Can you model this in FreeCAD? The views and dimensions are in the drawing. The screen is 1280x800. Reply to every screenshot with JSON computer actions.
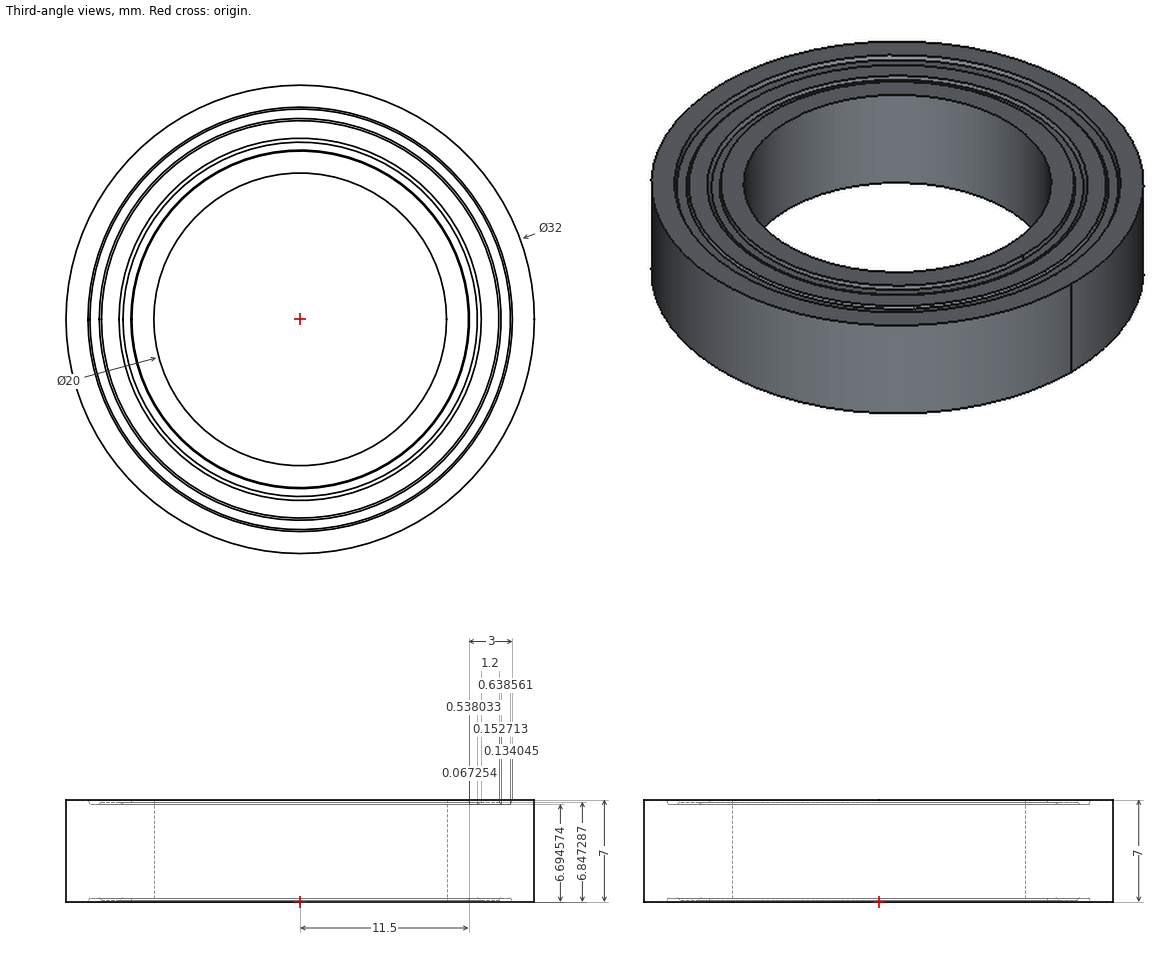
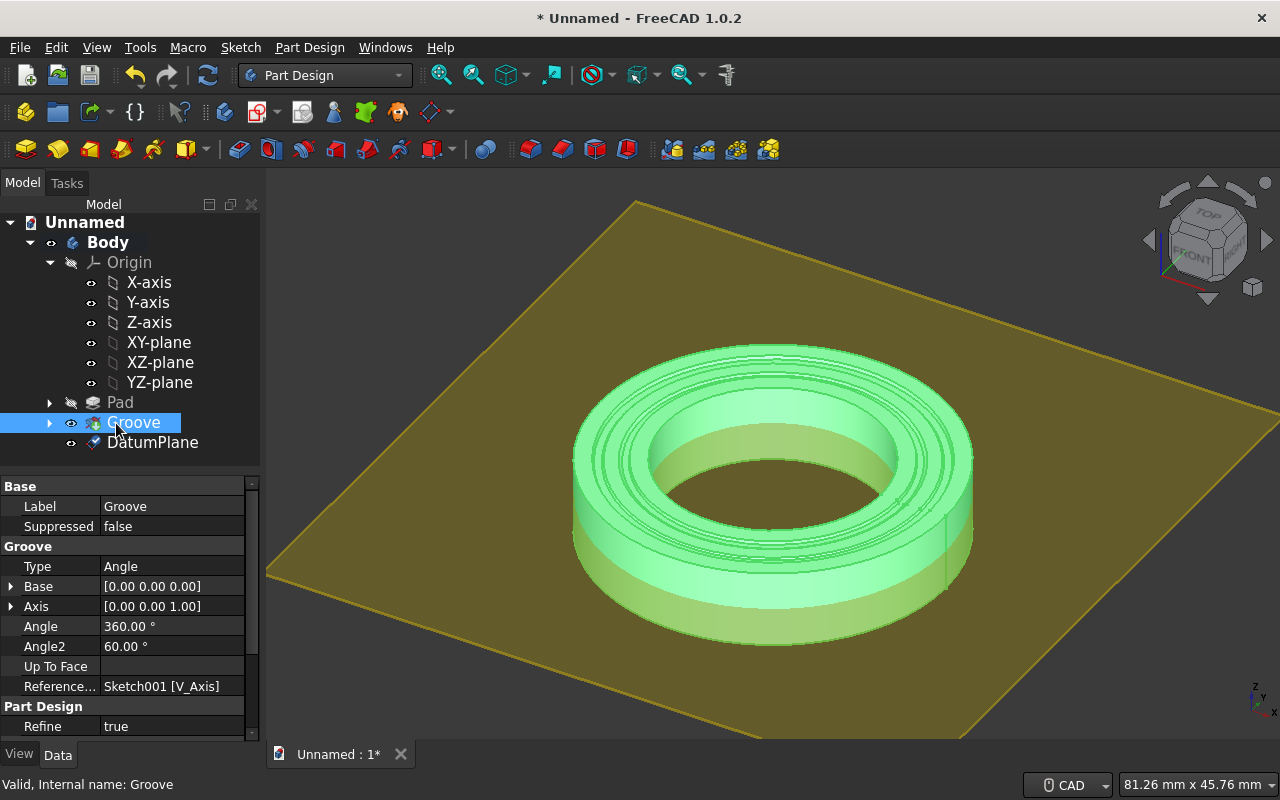
{"action": "left_click", "coordinate": [672, 150]}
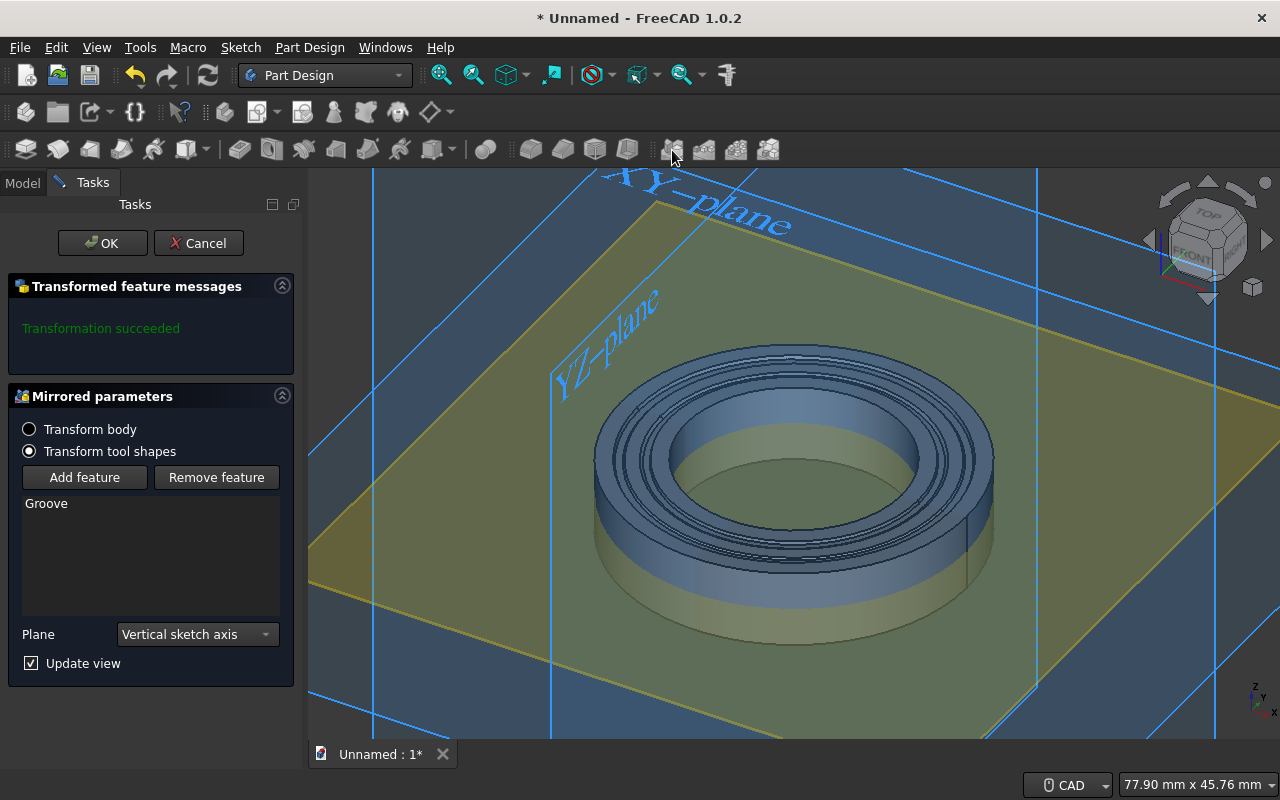
{"action": "left_click", "coordinate": [198, 634]}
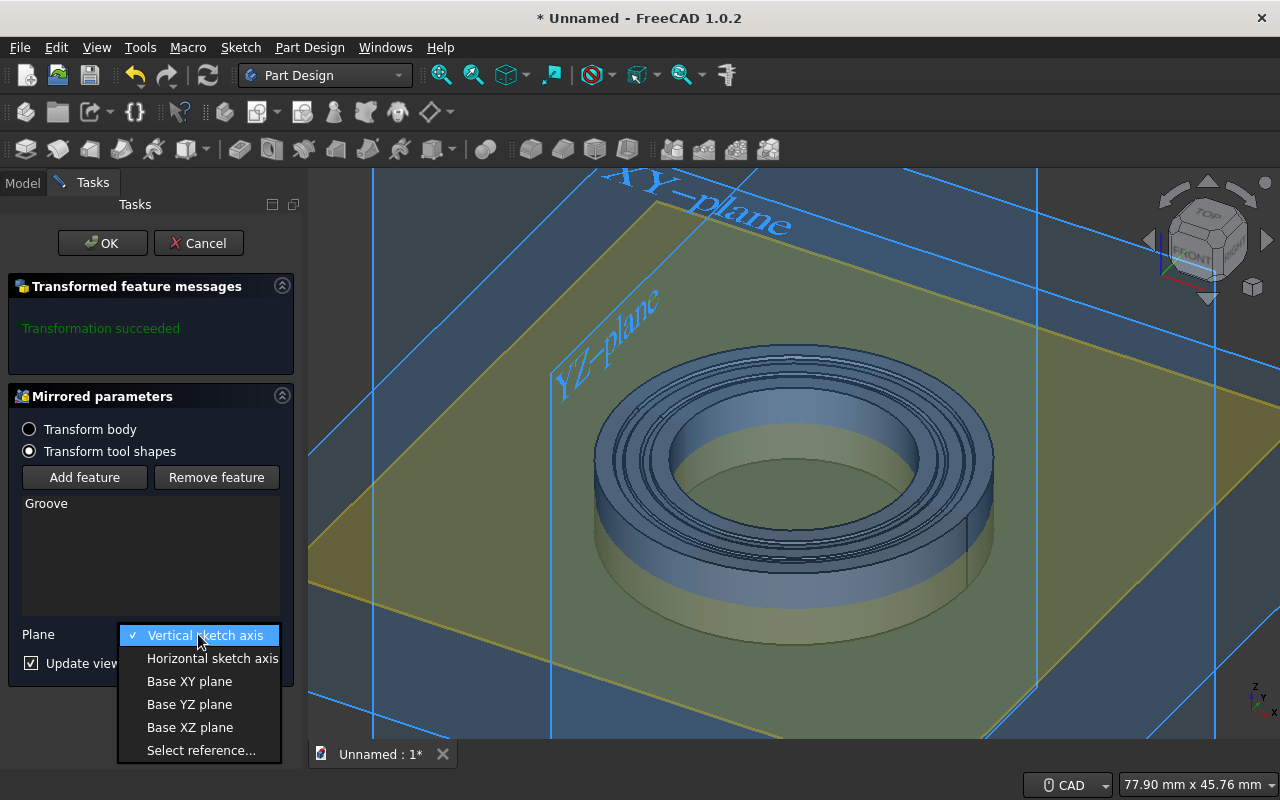
{"action": "left_click", "coordinate": [198, 750]}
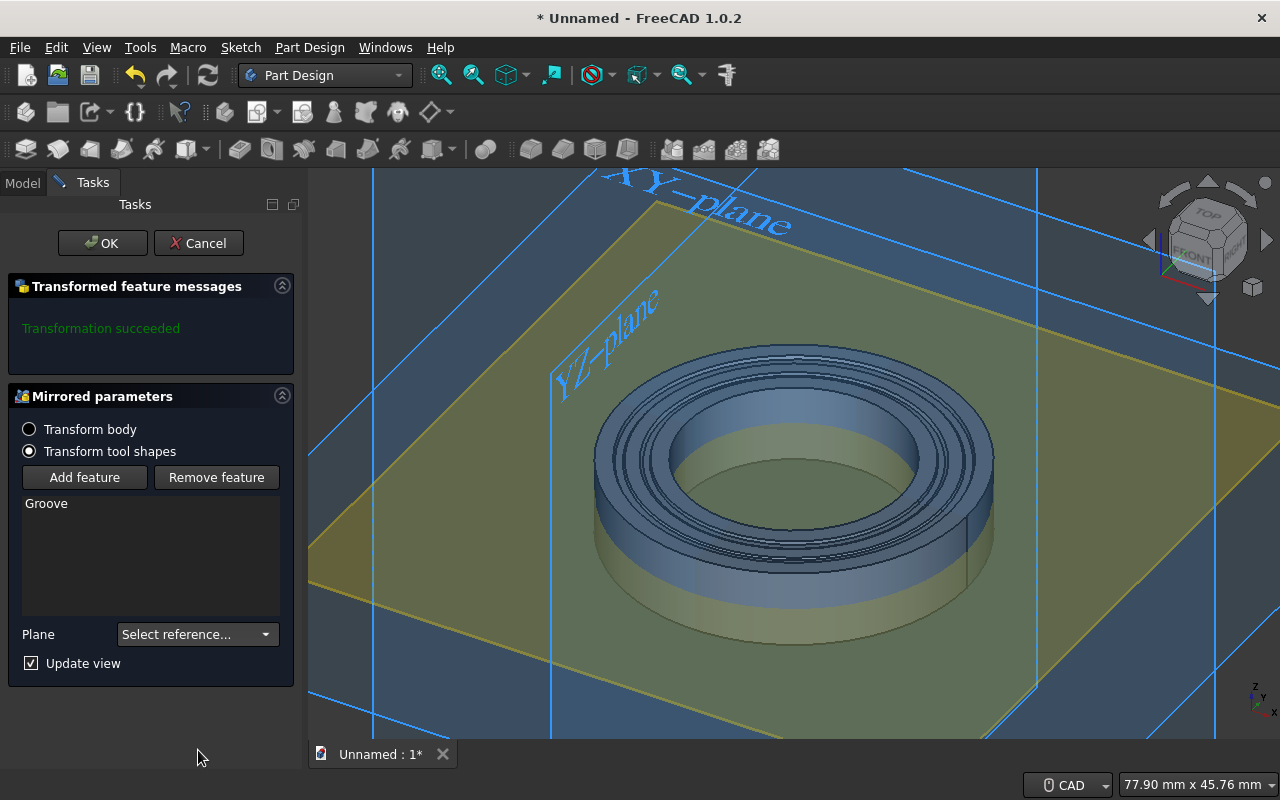
{"action": "left_click", "coordinate": [23, 182]}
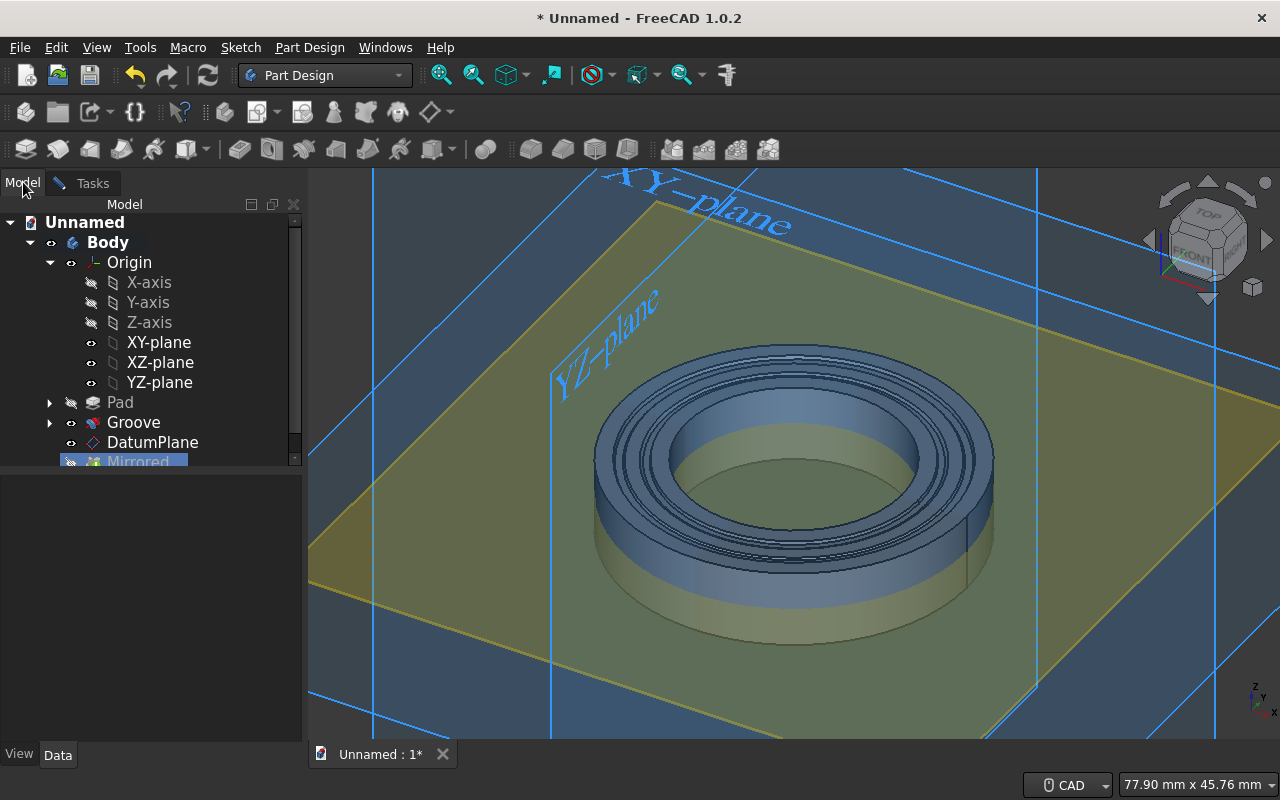
{"action": "left_click", "coordinate": [116, 443]}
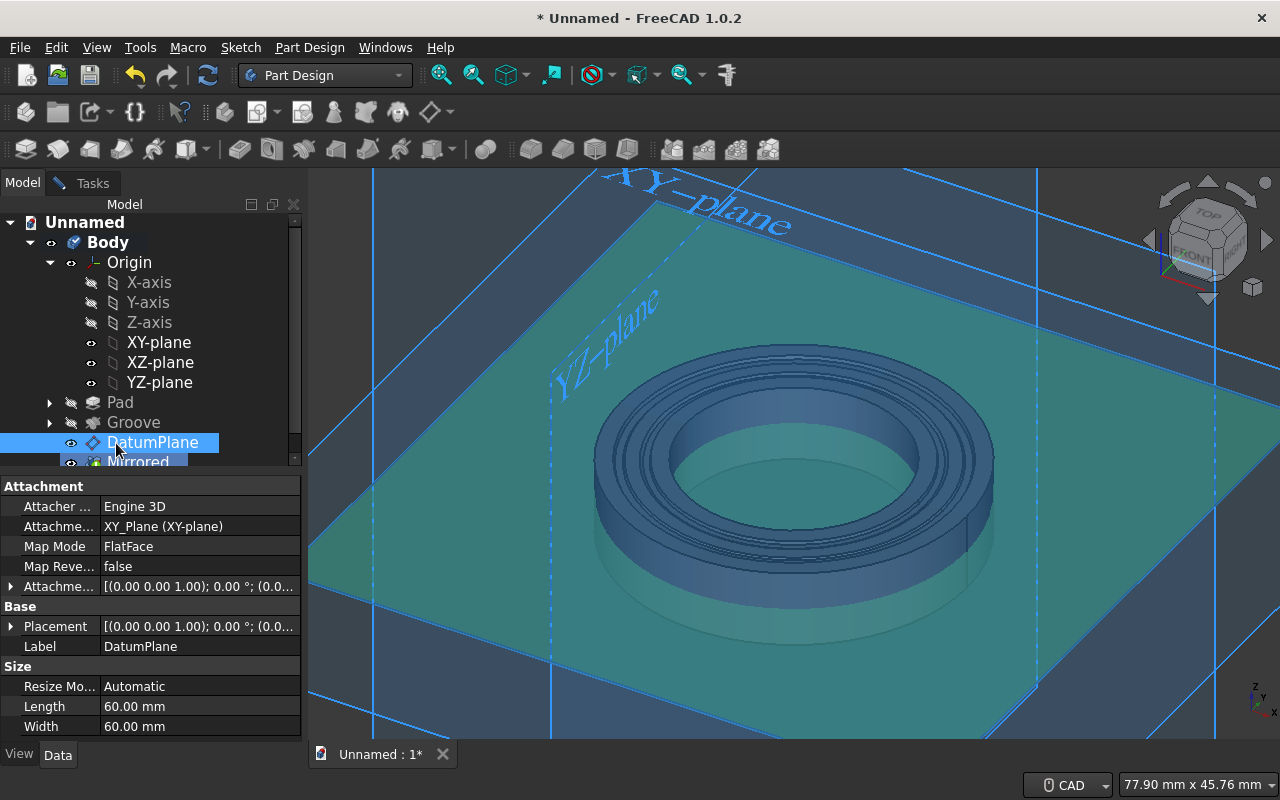
{"action": "left_click", "coordinate": [84, 182]}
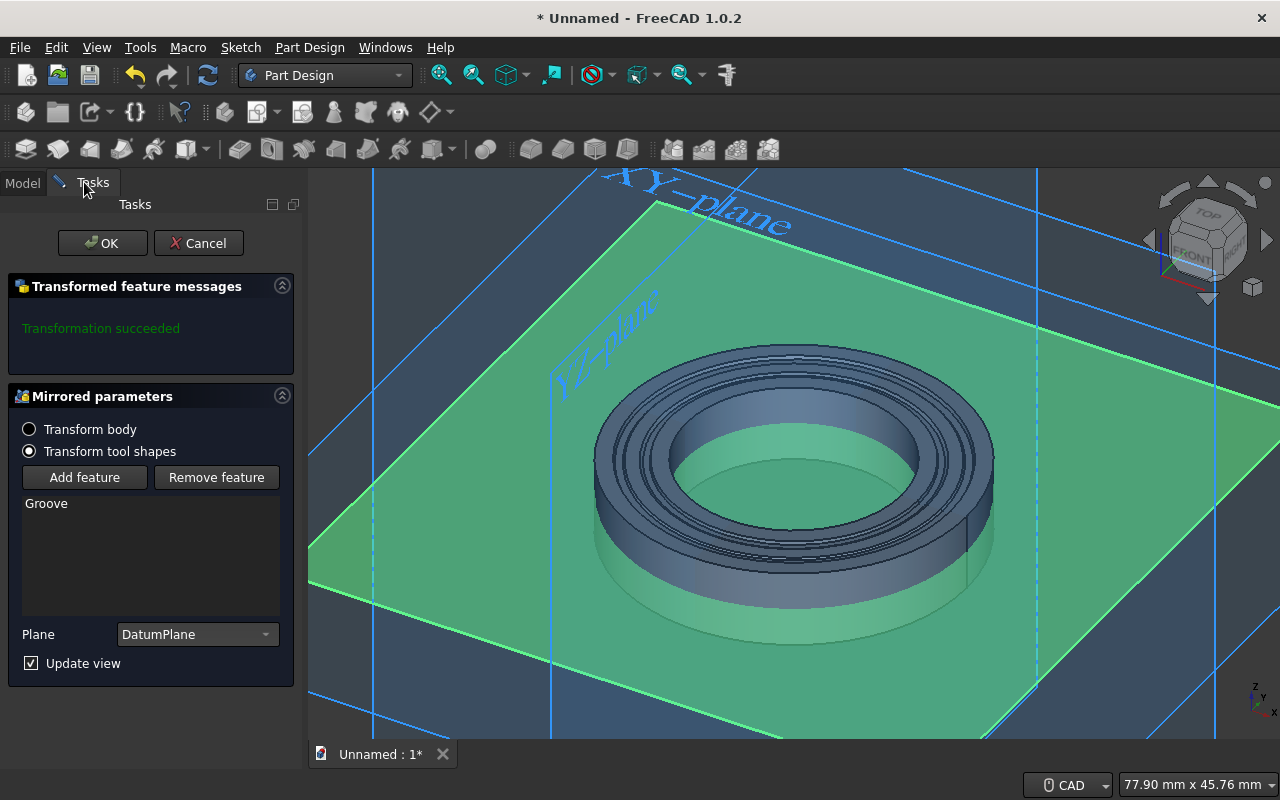
{"action": "left_click", "coordinate": [103, 243]}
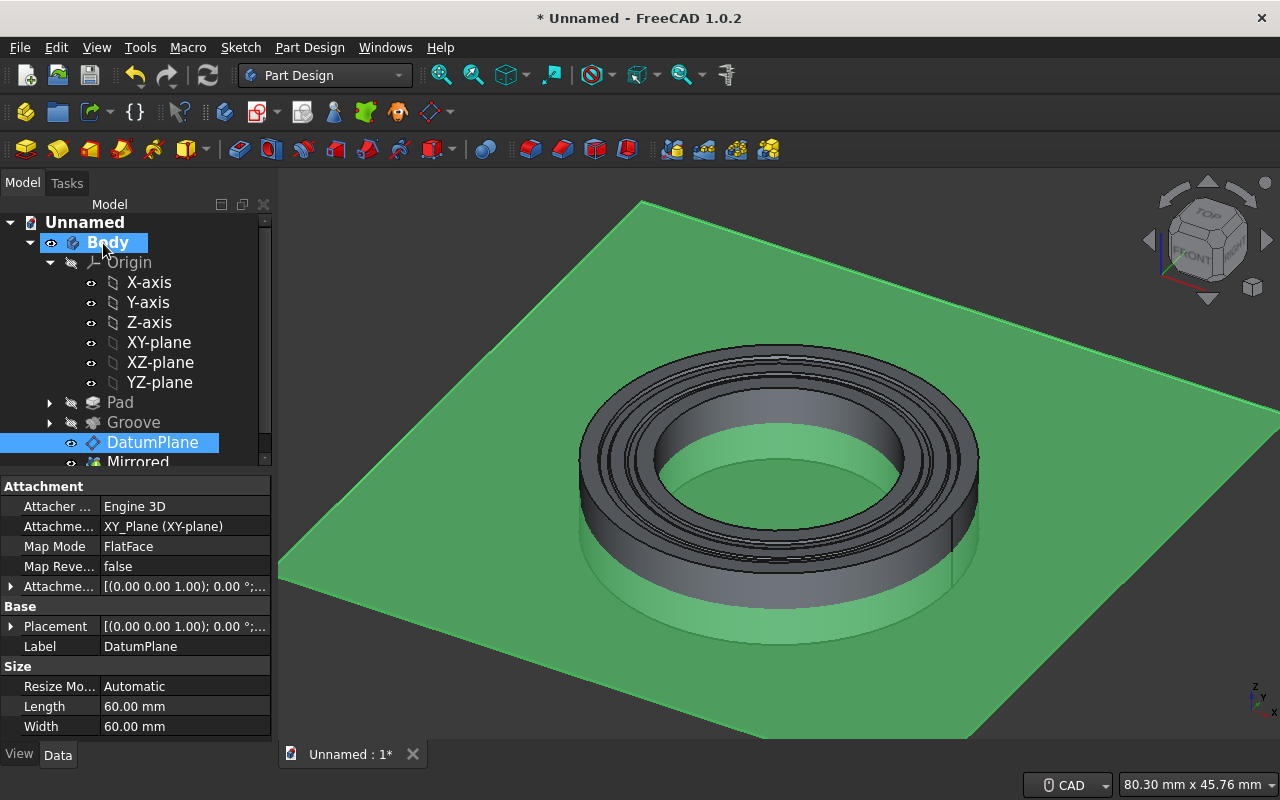
{"action": "left_click", "coordinate": [116, 443]}
{"action": "key", "text": "space"}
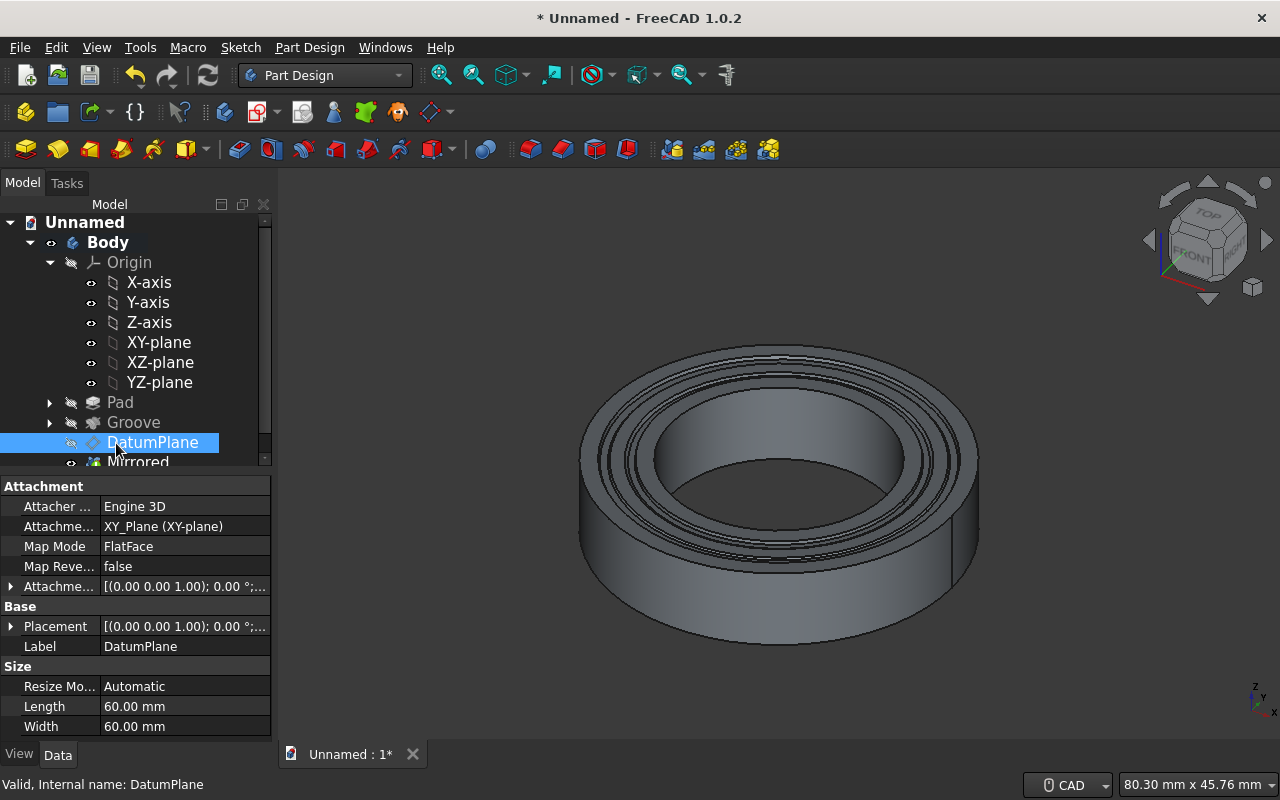
{"action": "key", "text": "0"}